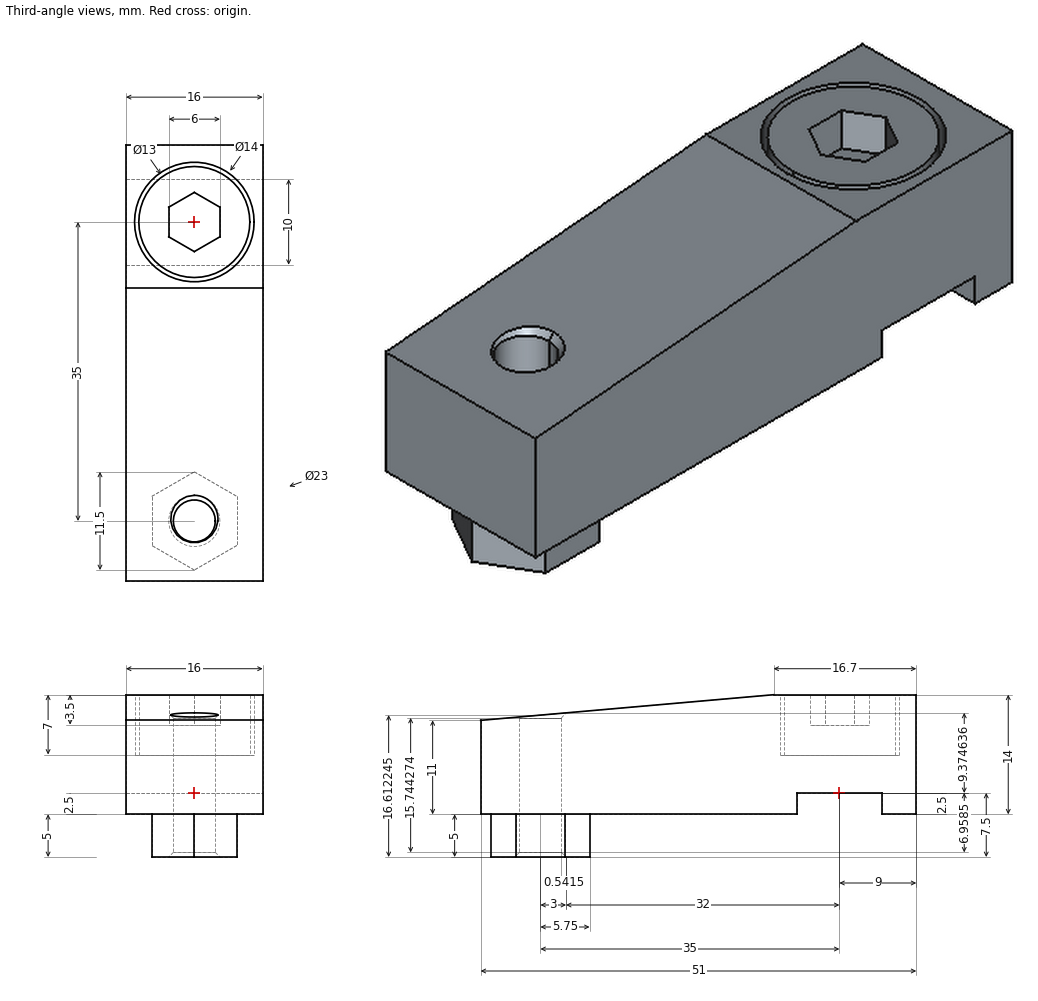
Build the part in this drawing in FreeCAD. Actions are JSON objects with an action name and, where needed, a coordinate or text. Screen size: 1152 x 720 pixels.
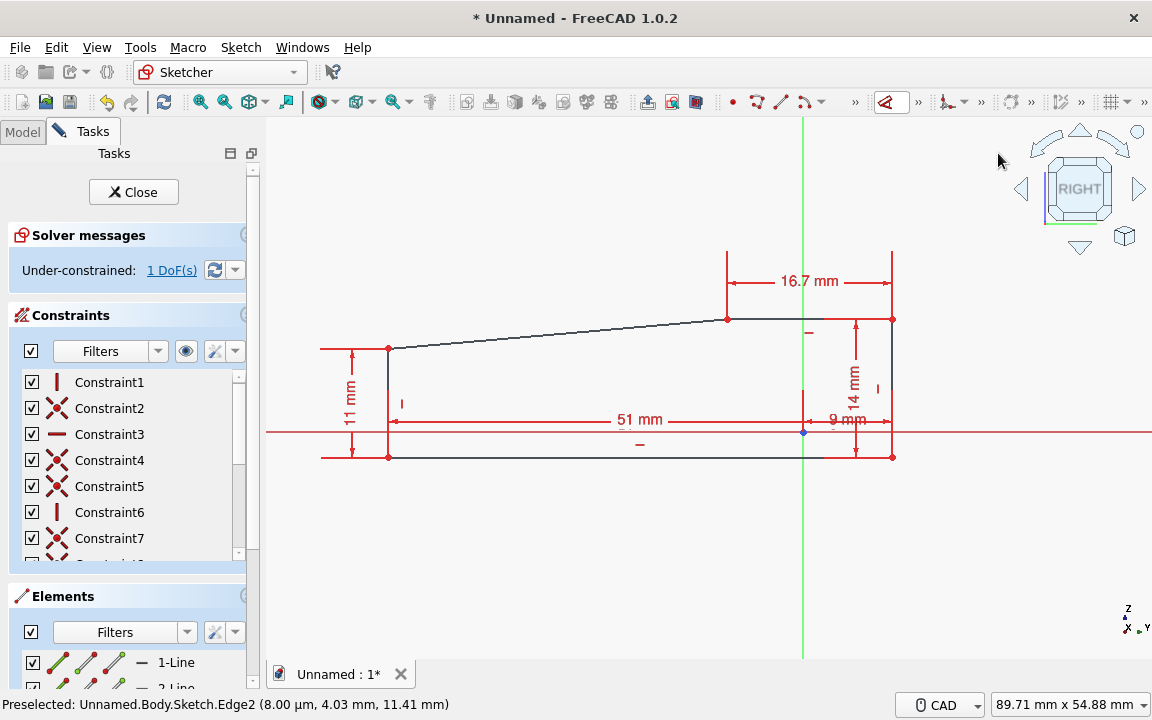
{"action": "scroll", "coordinate": [892, 458], "scroll_direction": "up", "scroll_amount": 3}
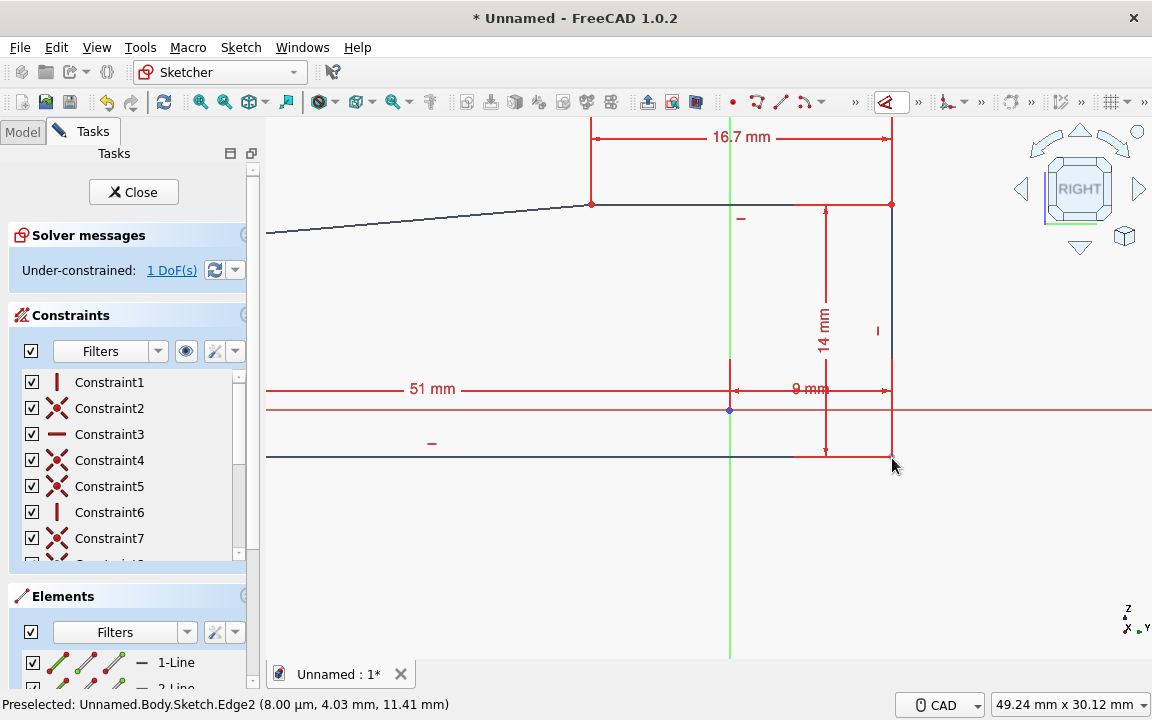
{"action": "left_click", "coordinate": [892, 457]}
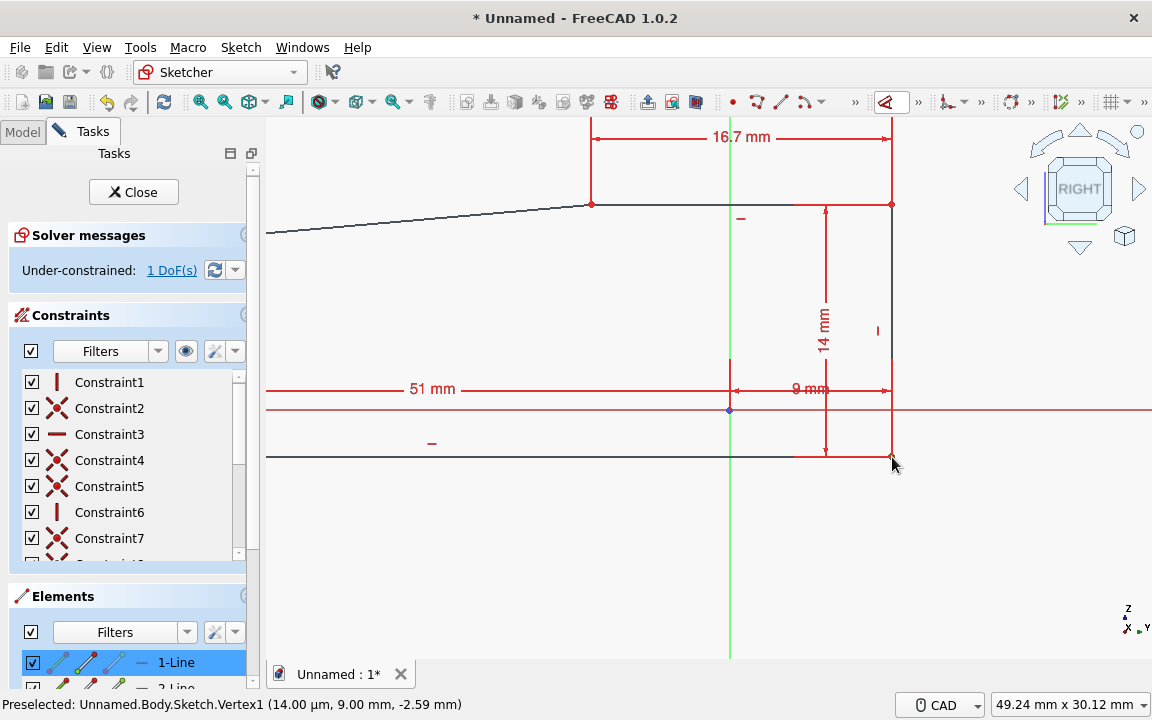
{"action": "key", "text": "i"}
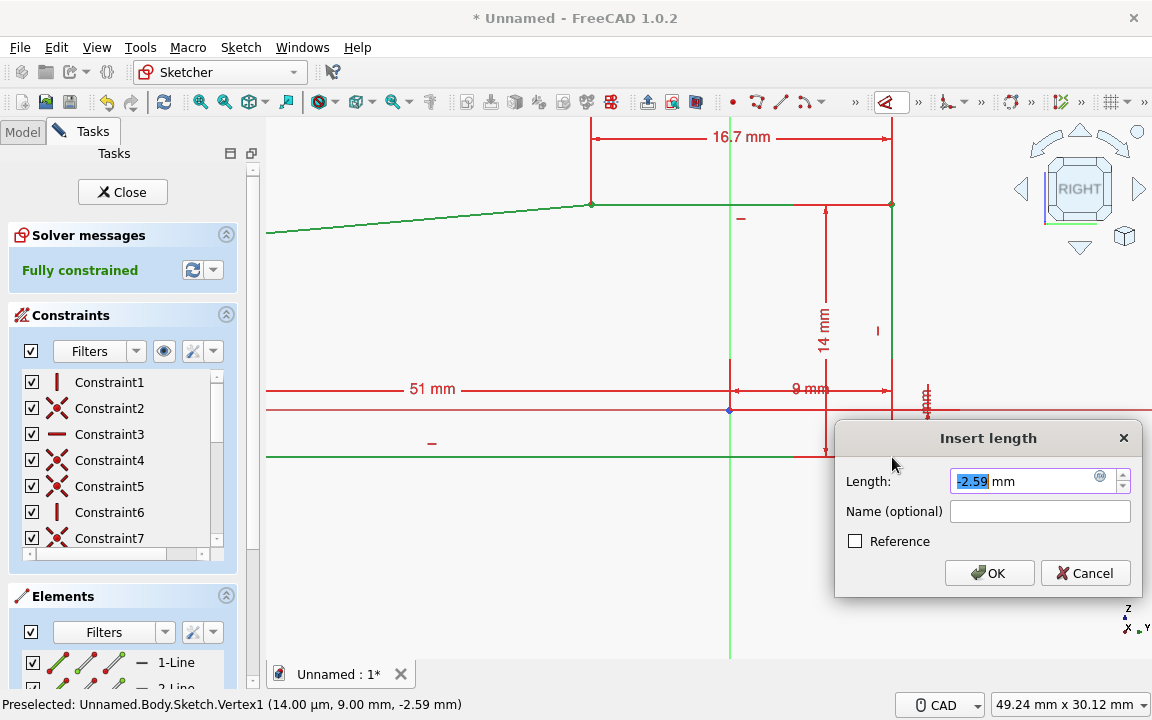
{"action": "type", "text": "-2.5"}
{"action": "key", "text": "Return"}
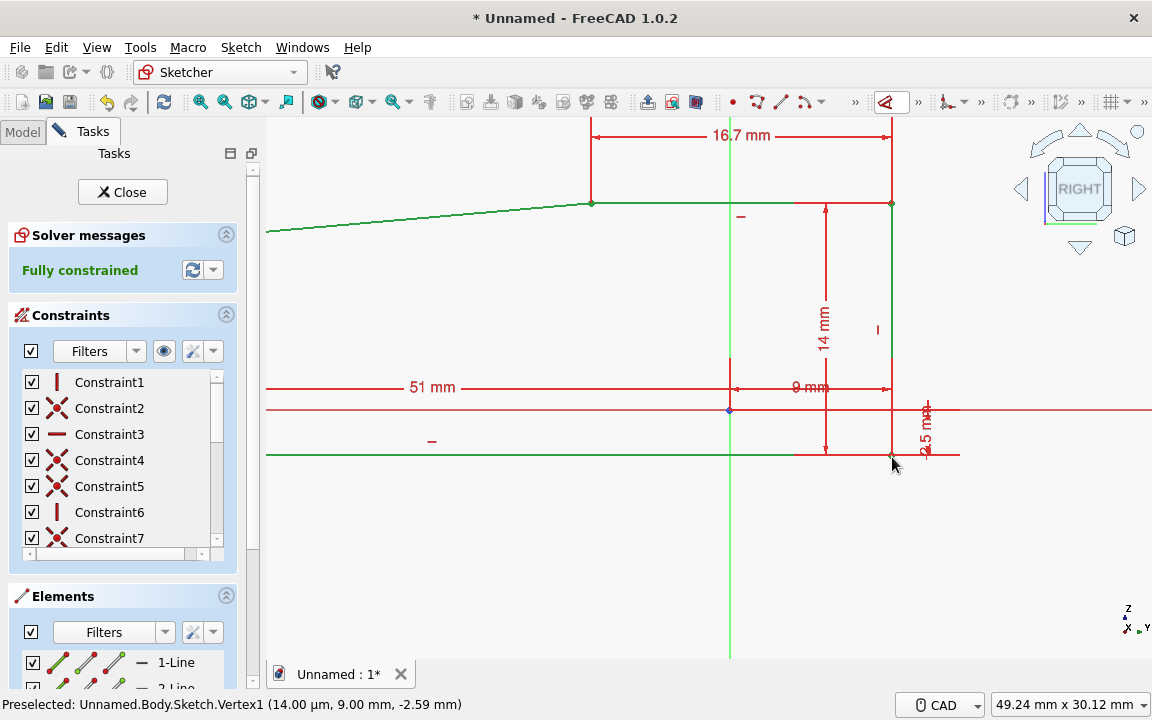
{"action": "left_click", "coordinate": [123, 192]}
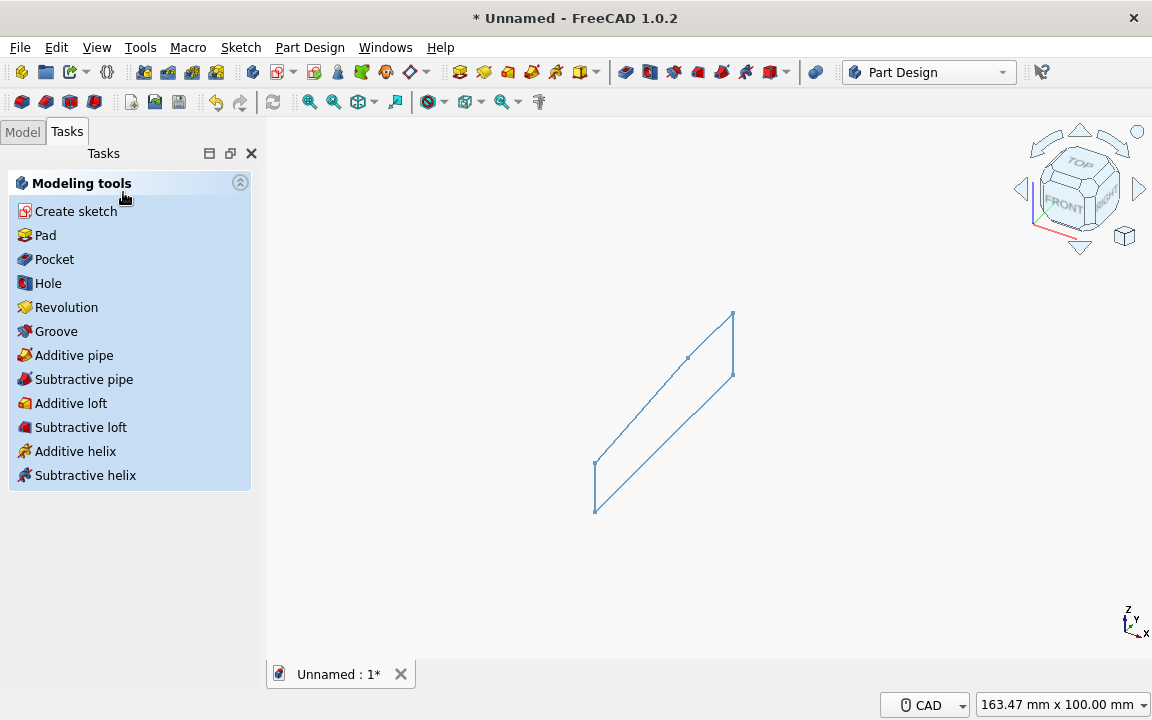
{"action": "left_click", "coordinate": [460, 72]}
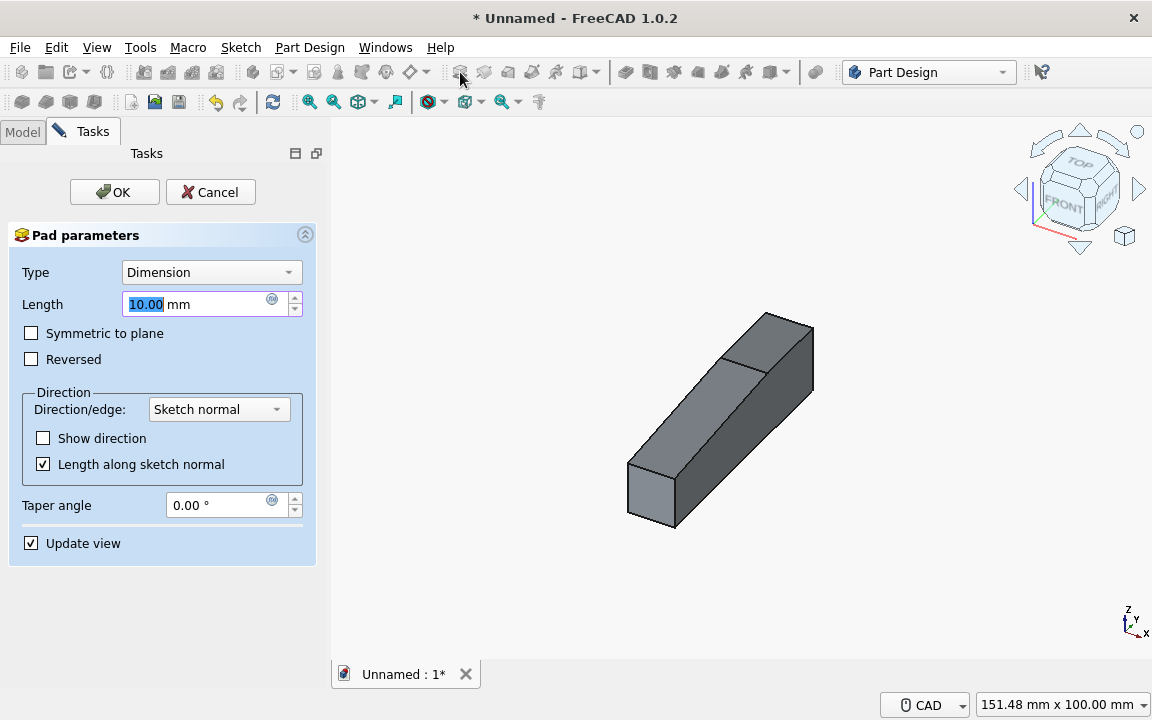
{"action": "type", "text": "16"}
{"action": "key", "text": "Tab"}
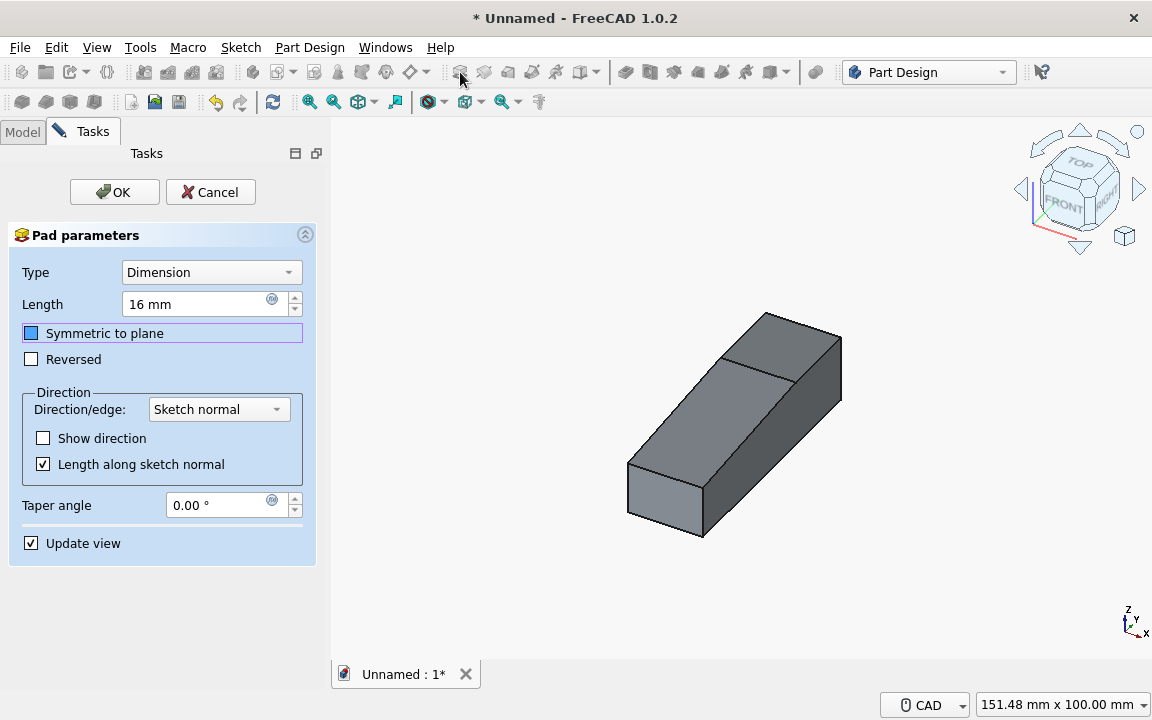
{"action": "left_click", "coordinate": [30, 333]}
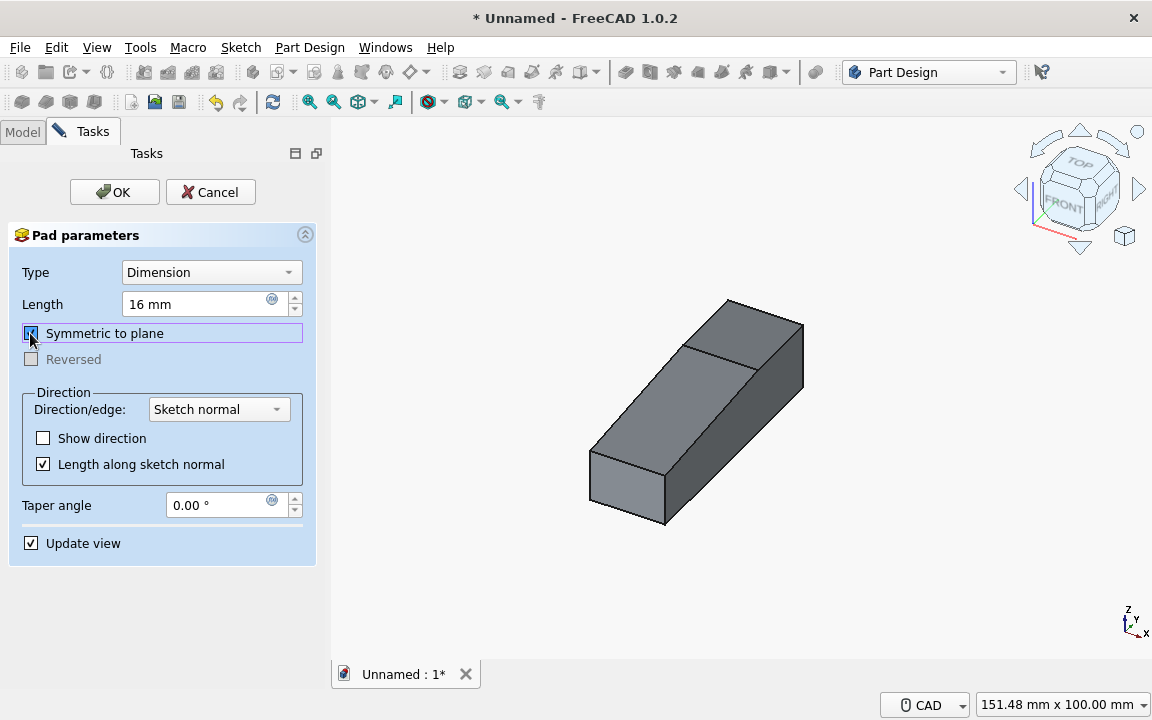
{"action": "left_click", "coordinate": [115, 192]}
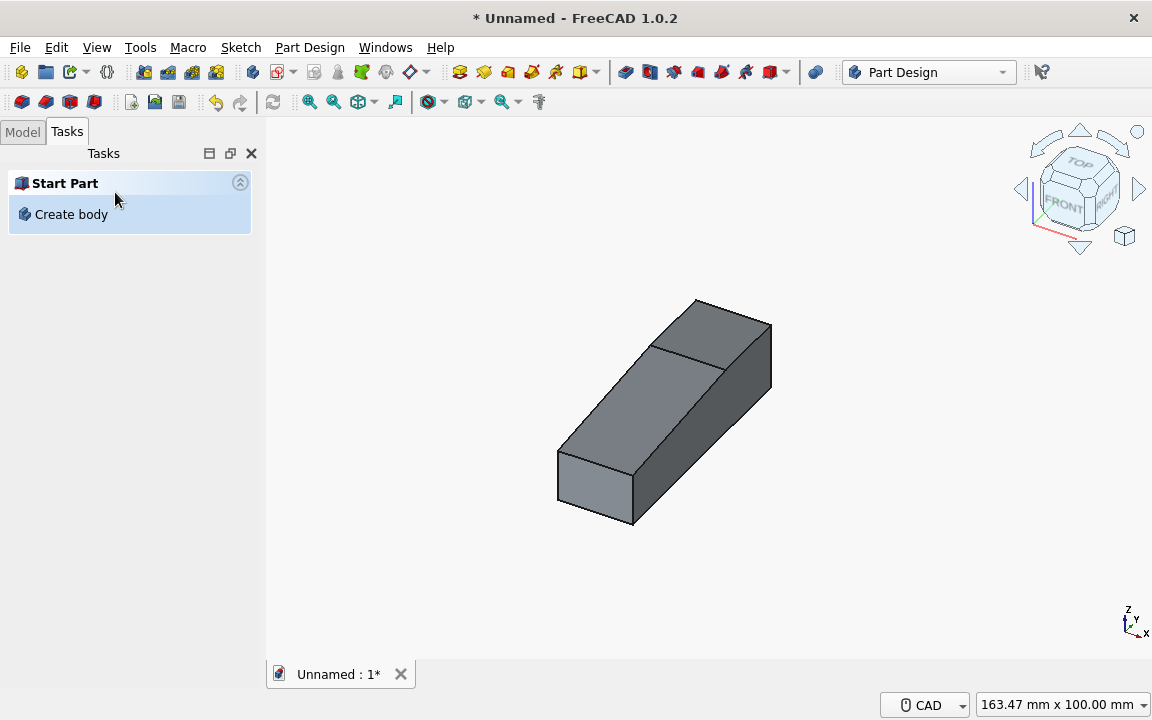
{"action": "left_click", "coordinate": [310, 102]}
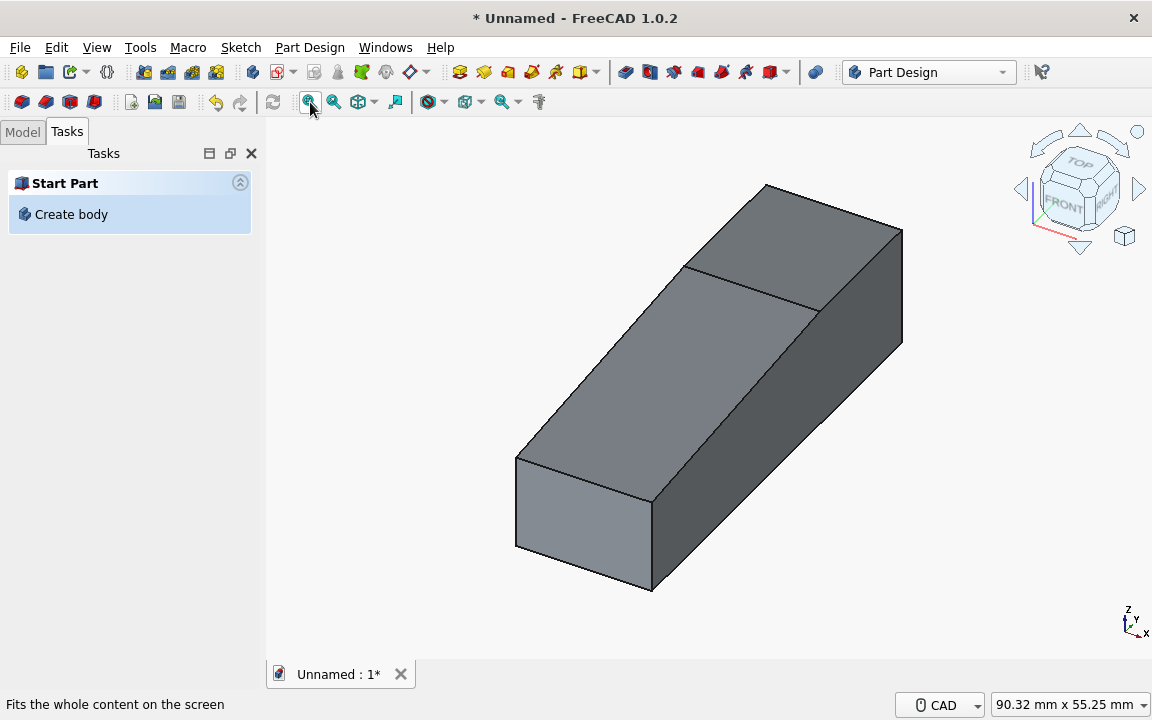
{"action": "left_click", "coordinate": [278, 72]}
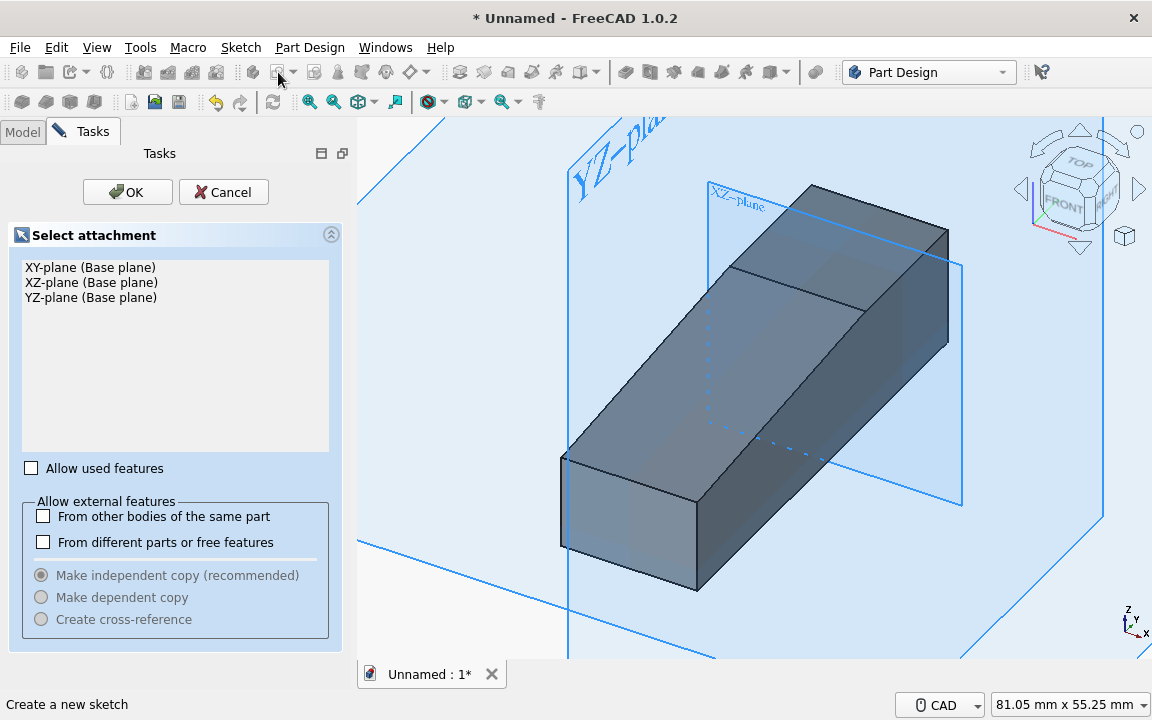
{"action": "left_click", "coordinate": [82, 268]}